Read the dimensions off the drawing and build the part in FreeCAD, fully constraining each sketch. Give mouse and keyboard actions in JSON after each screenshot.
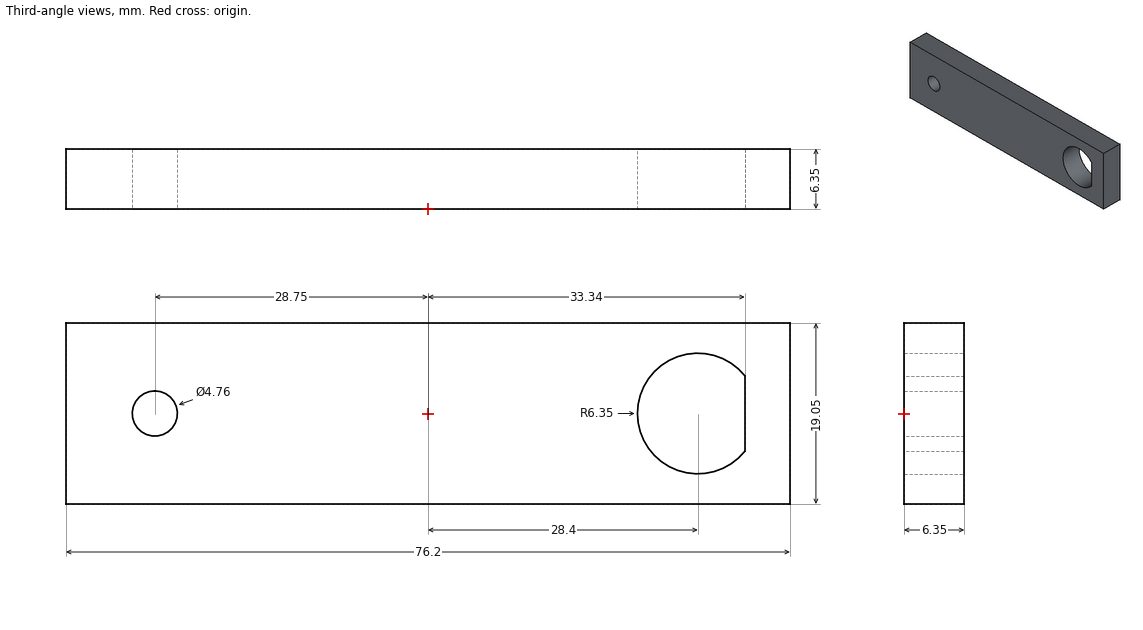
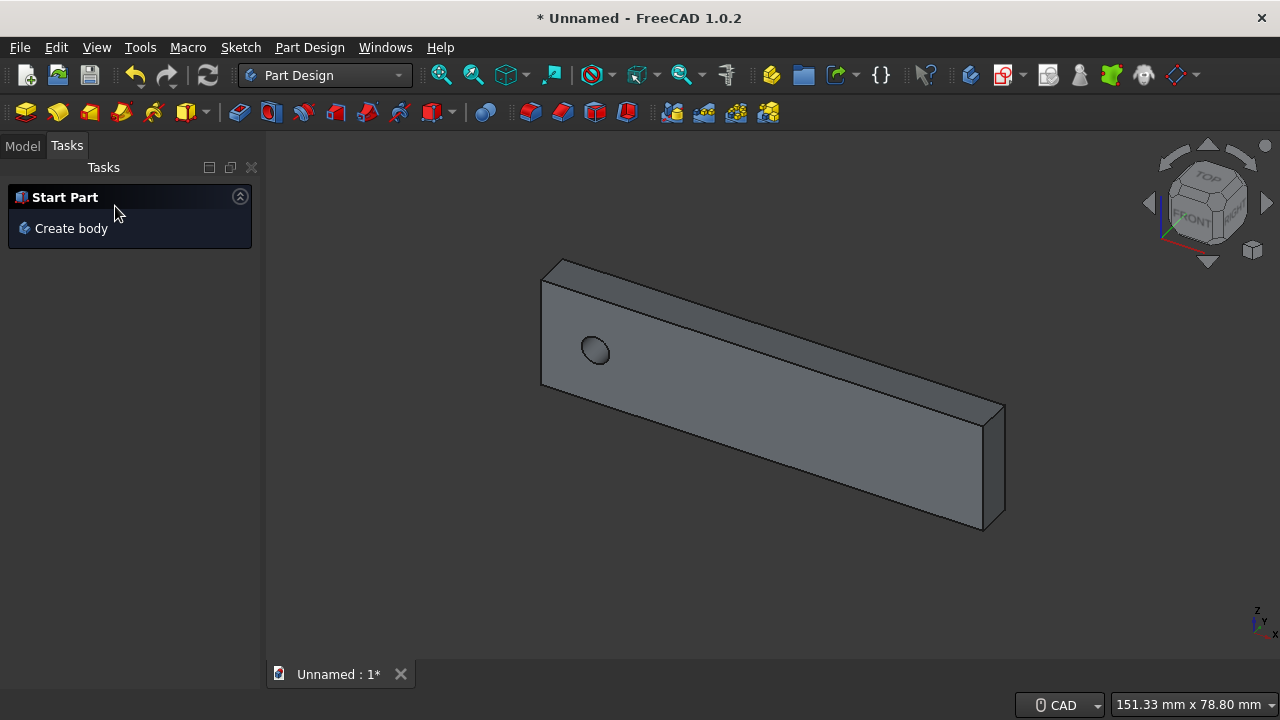
{"action": "key", "text": "4"}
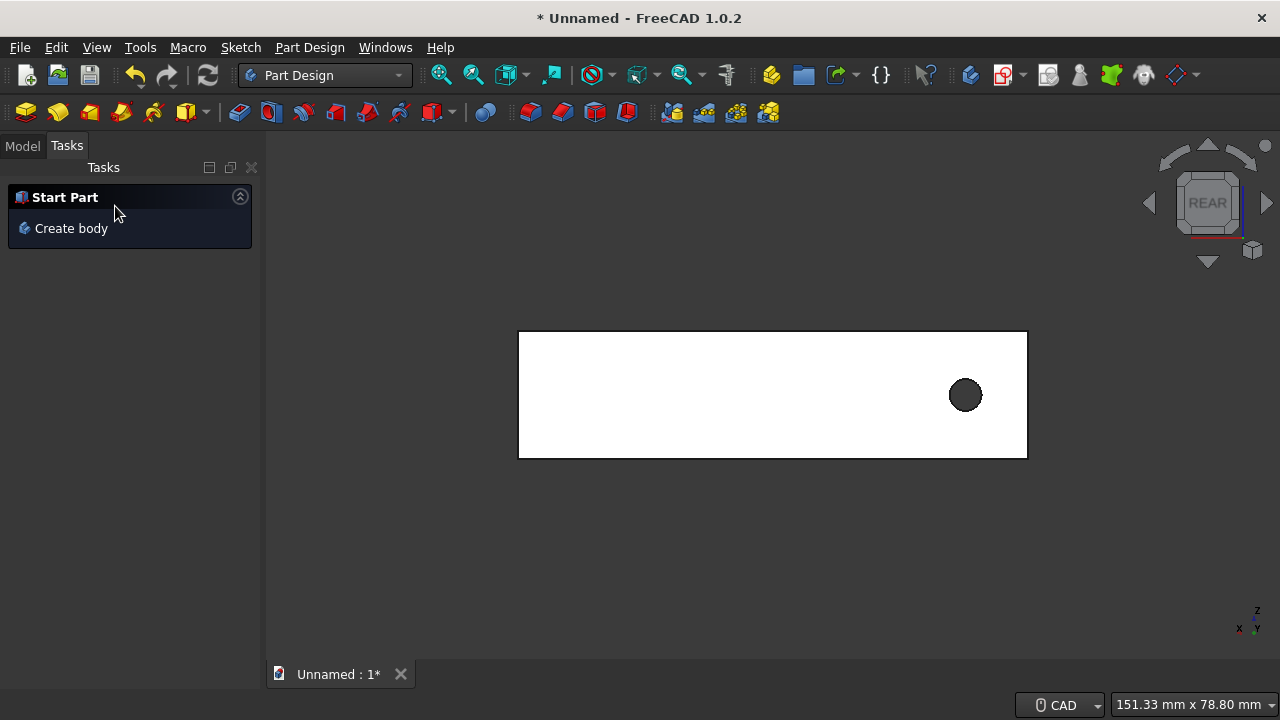
{"action": "left_click", "coordinate": [627, 394]}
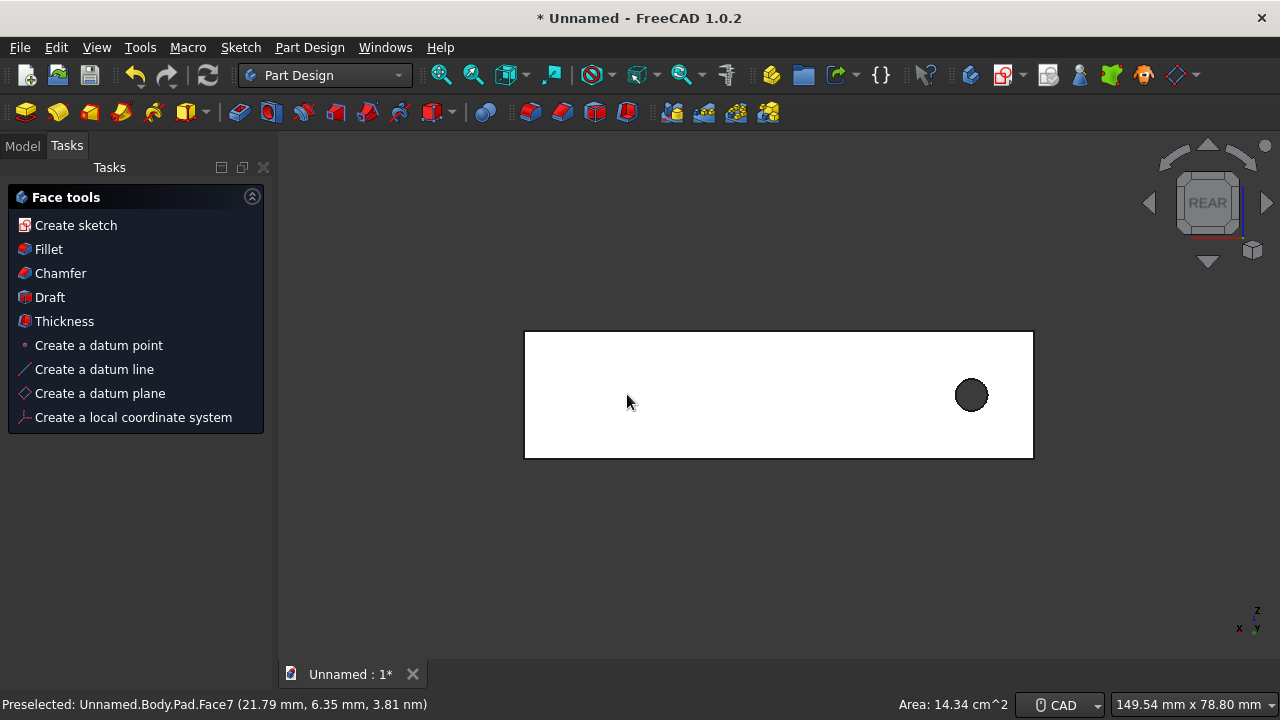
{"action": "left_click", "coordinate": [1004, 76]}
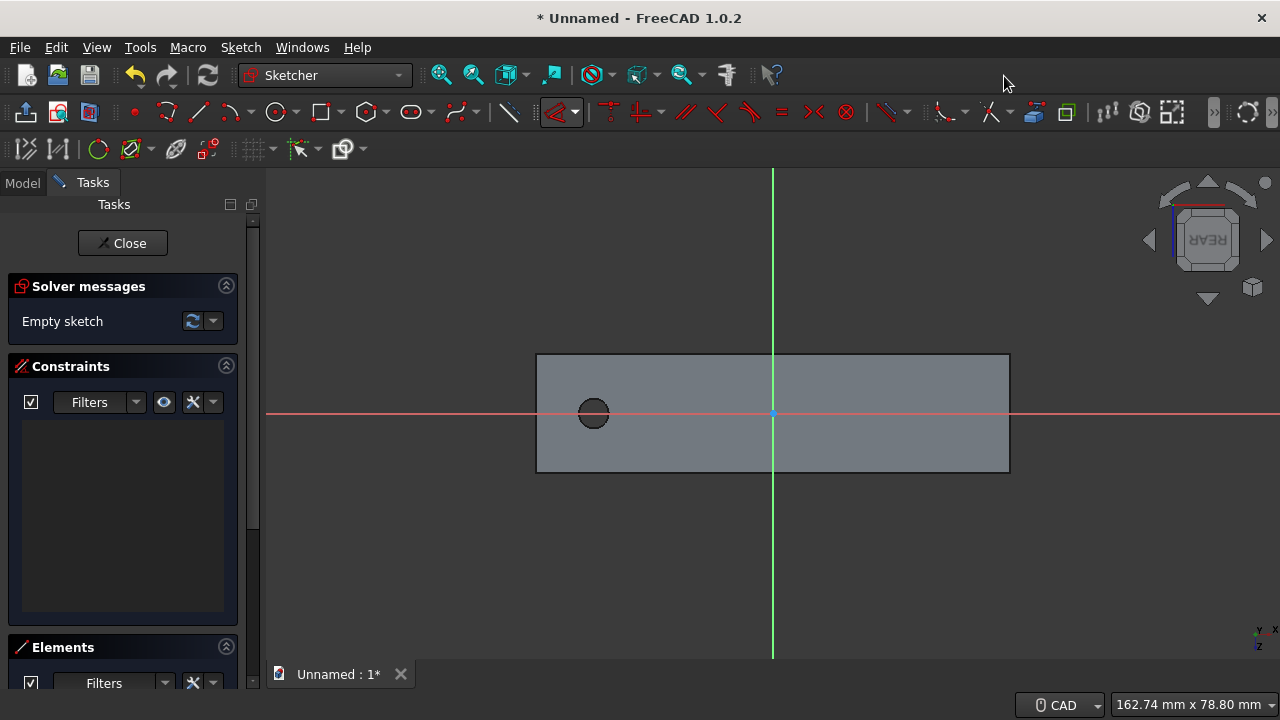
{"action": "scroll", "coordinate": [993, 413], "scroll_direction": "up", "scroll_amount": 9}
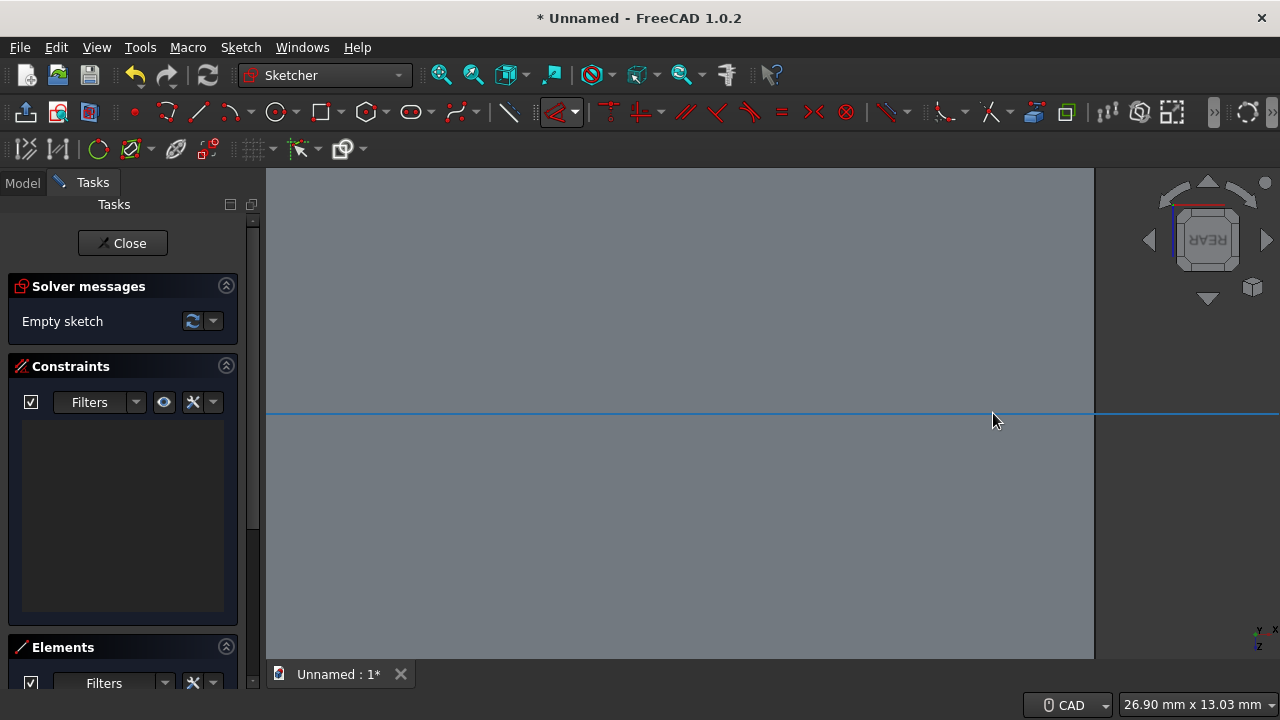
{"action": "key", "text": "g l"}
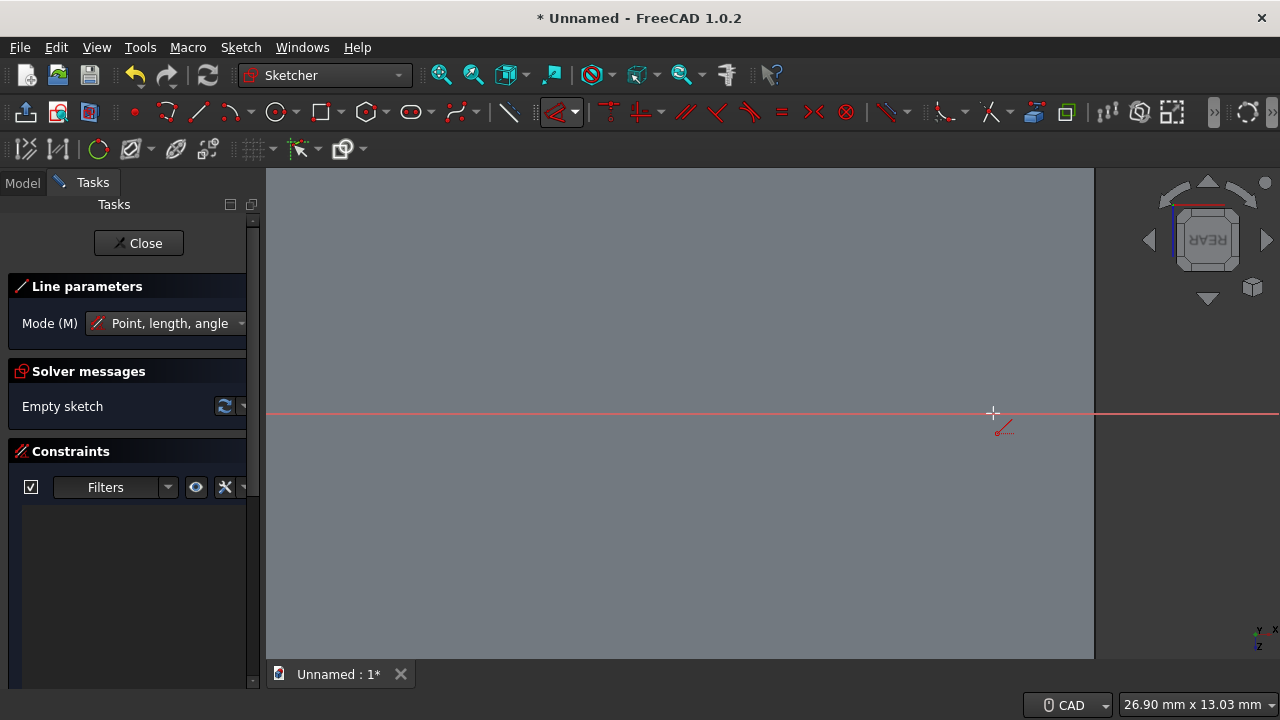
{"action": "left_click", "coordinate": [915, 564]}
{"action": "left_click", "coordinate": [915, 263]}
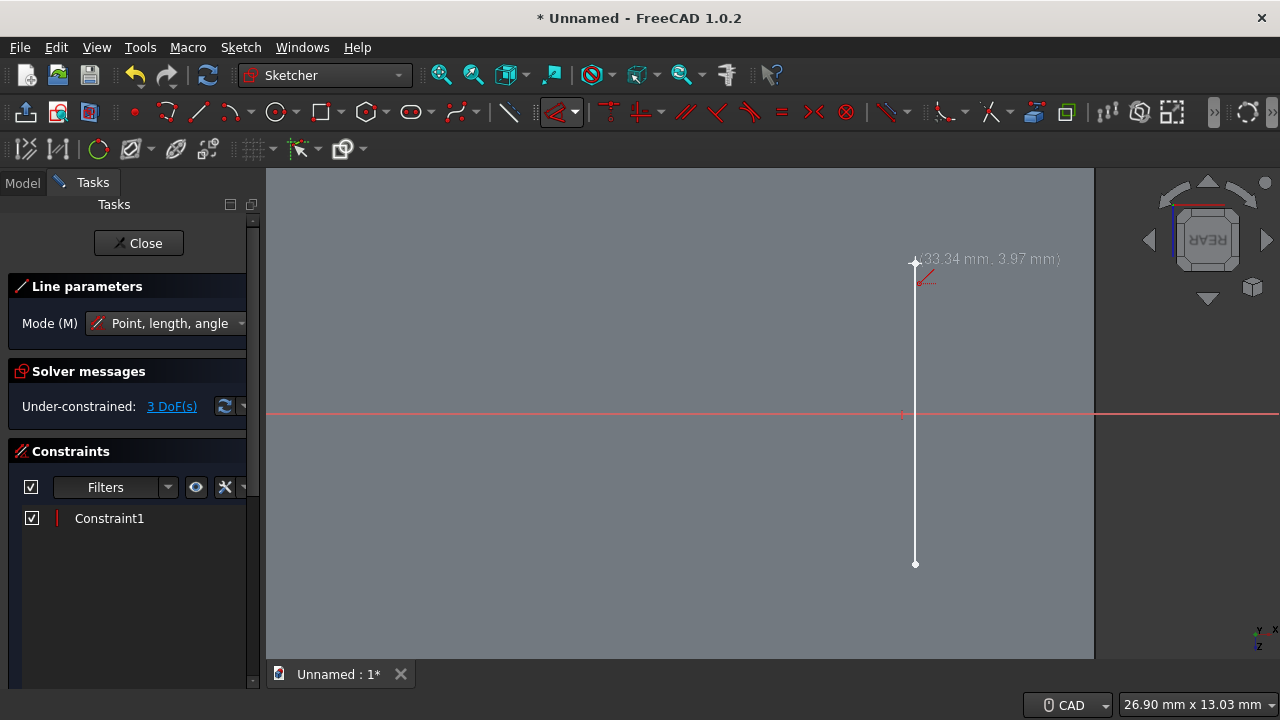
{"action": "key", "text": "g 3 a"}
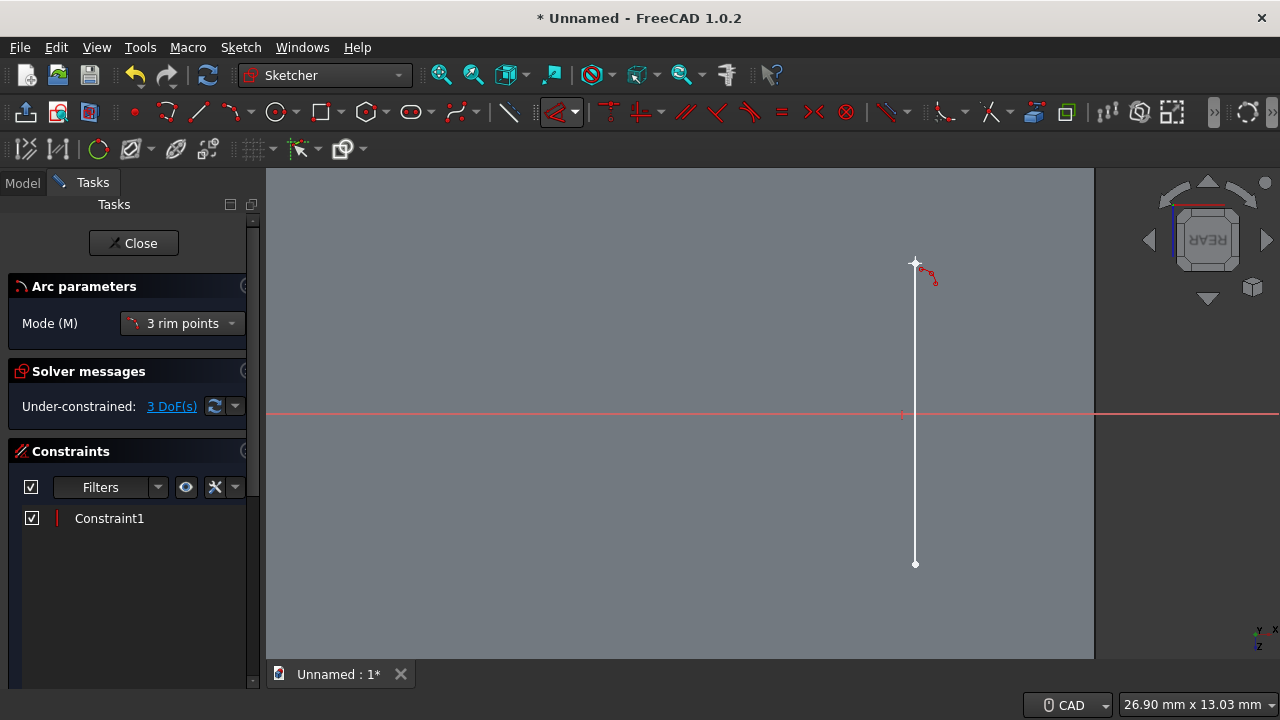
{"action": "left_click", "coordinate": [915, 264]}
{"action": "left_click", "coordinate": [915, 565]}
{"action": "left_click", "coordinate": [518, 300]}
{"action": "key", "text": "Escape"}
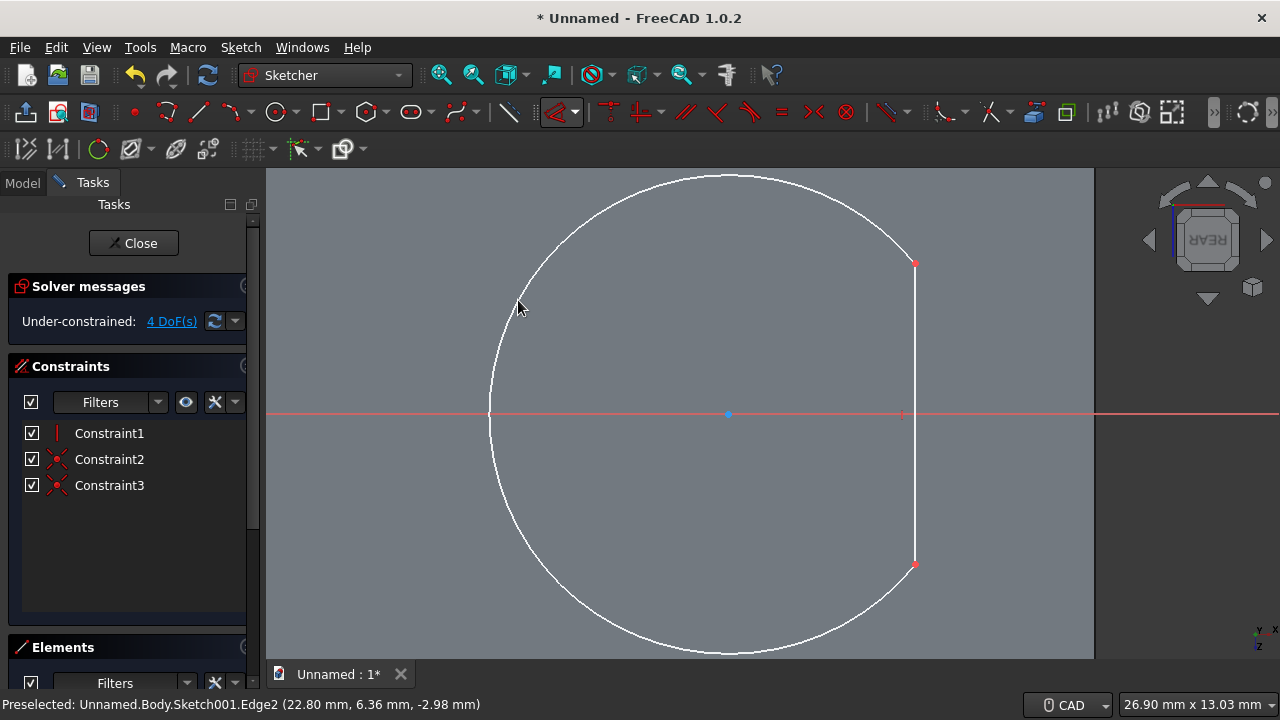
{"action": "left_click", "coordinate": [729, 414]}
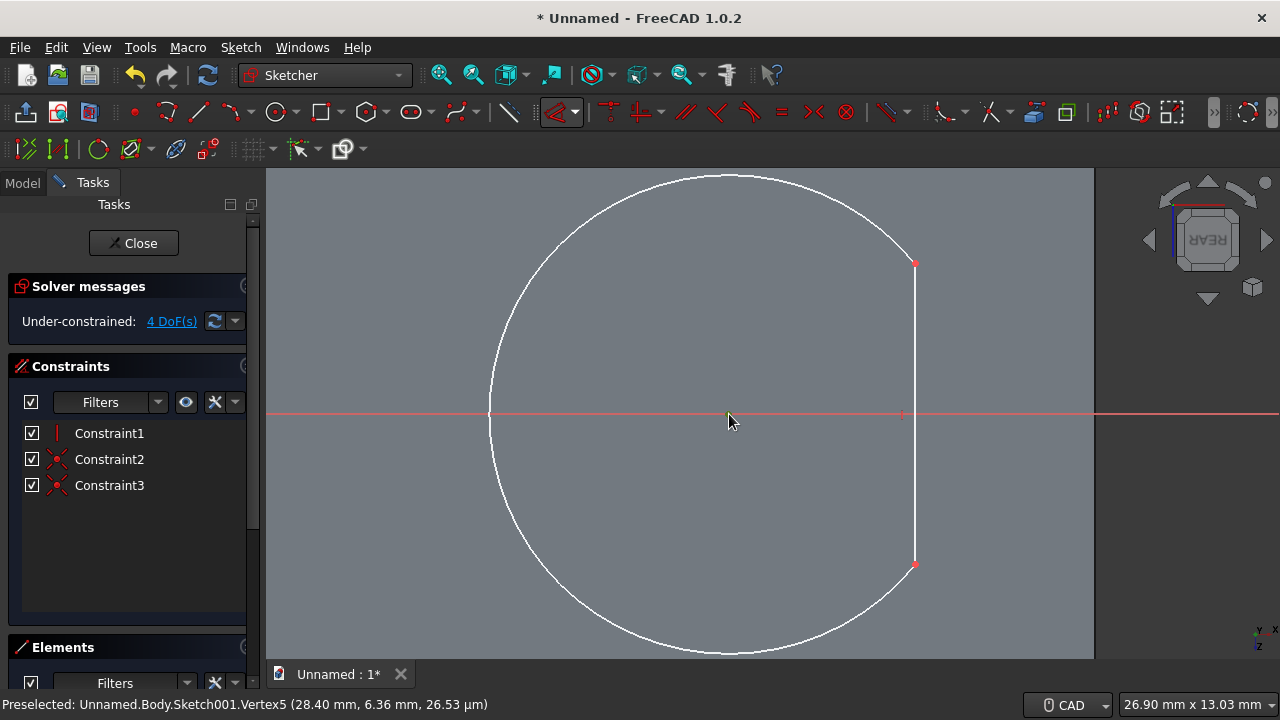
{"action": "left_click", "coordinate": [353, 413]}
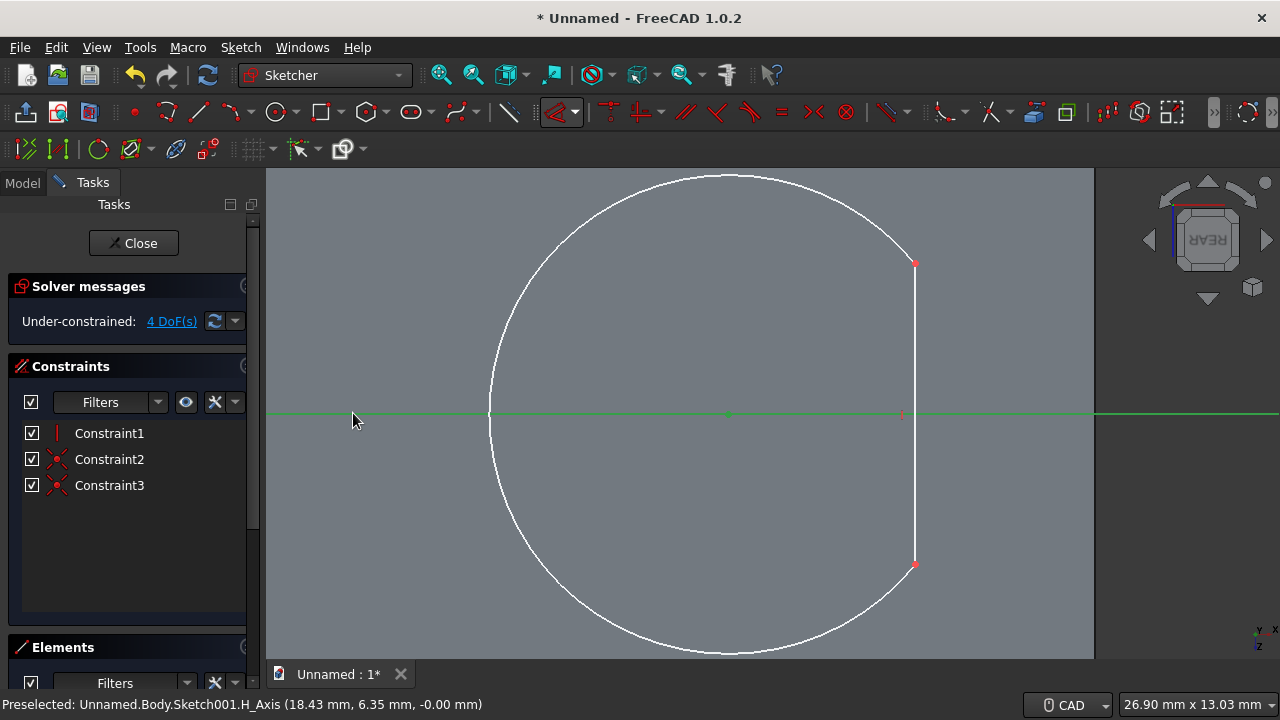
{"action": "key", "text": "c"}